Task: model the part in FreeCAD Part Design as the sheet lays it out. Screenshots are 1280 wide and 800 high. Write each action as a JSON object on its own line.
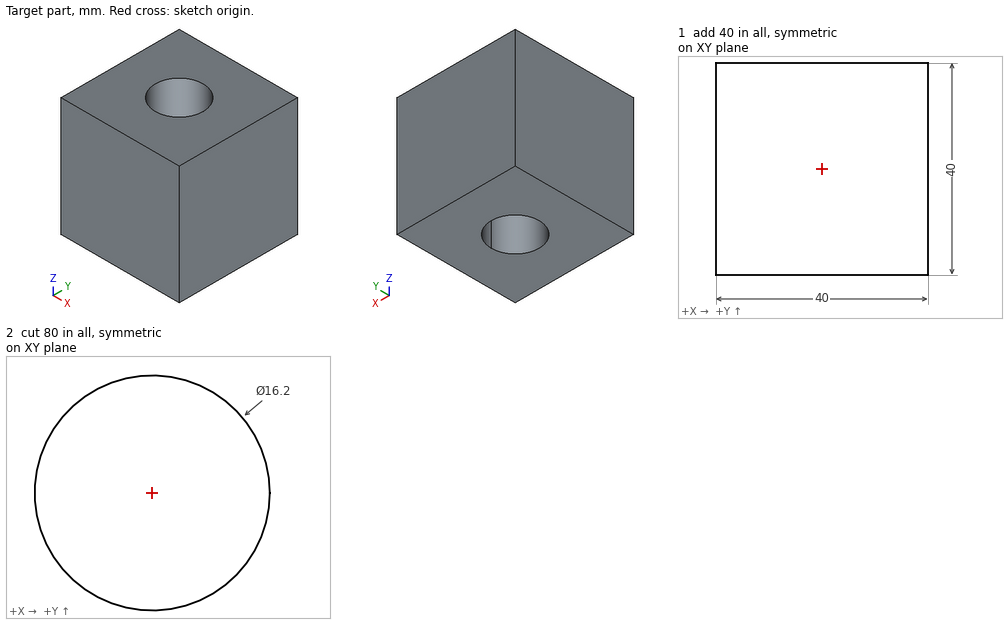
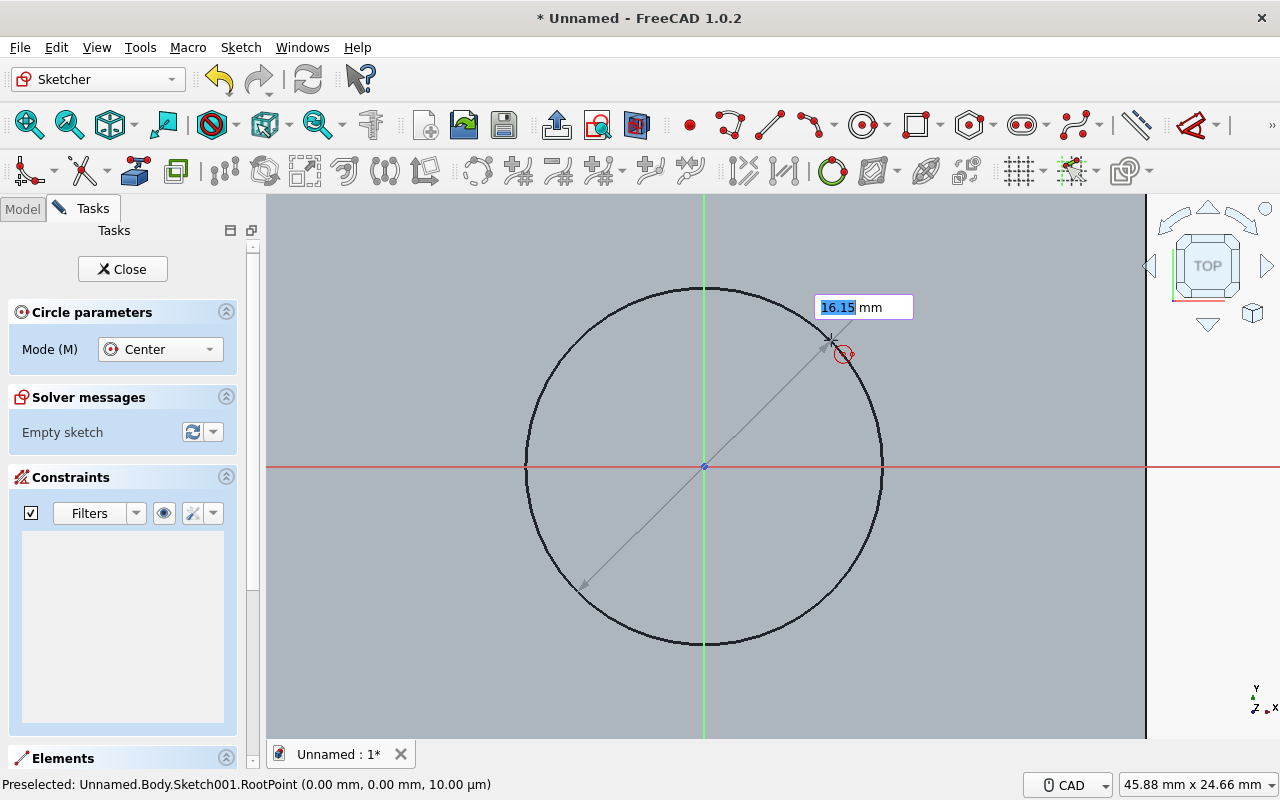
{"action": "type", "text": "16.2"}
{"action": "key", "text": "Return"}
{"action": "key", "text": "Escape"}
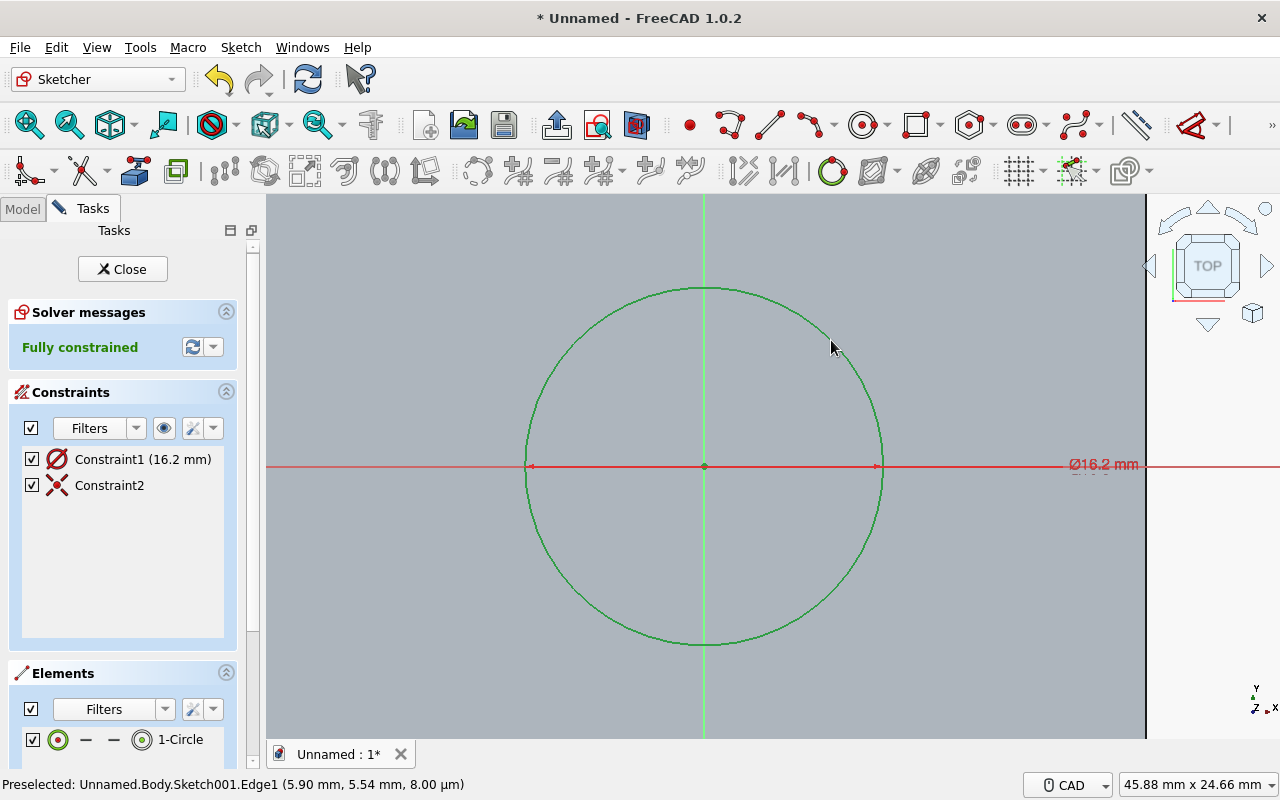
{"action": "left_click", "coordinate": [123, 269]}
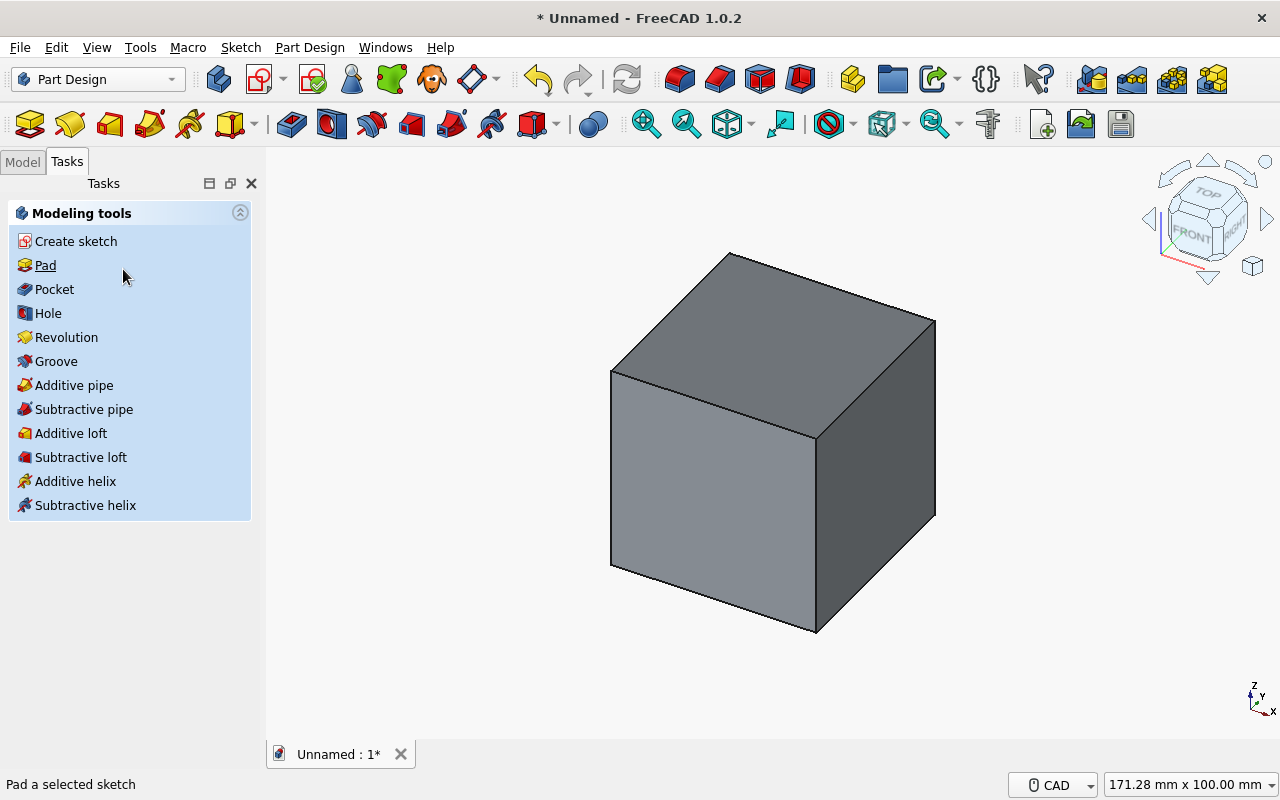
{"action": "left_click", "coordinate": [292, 124]}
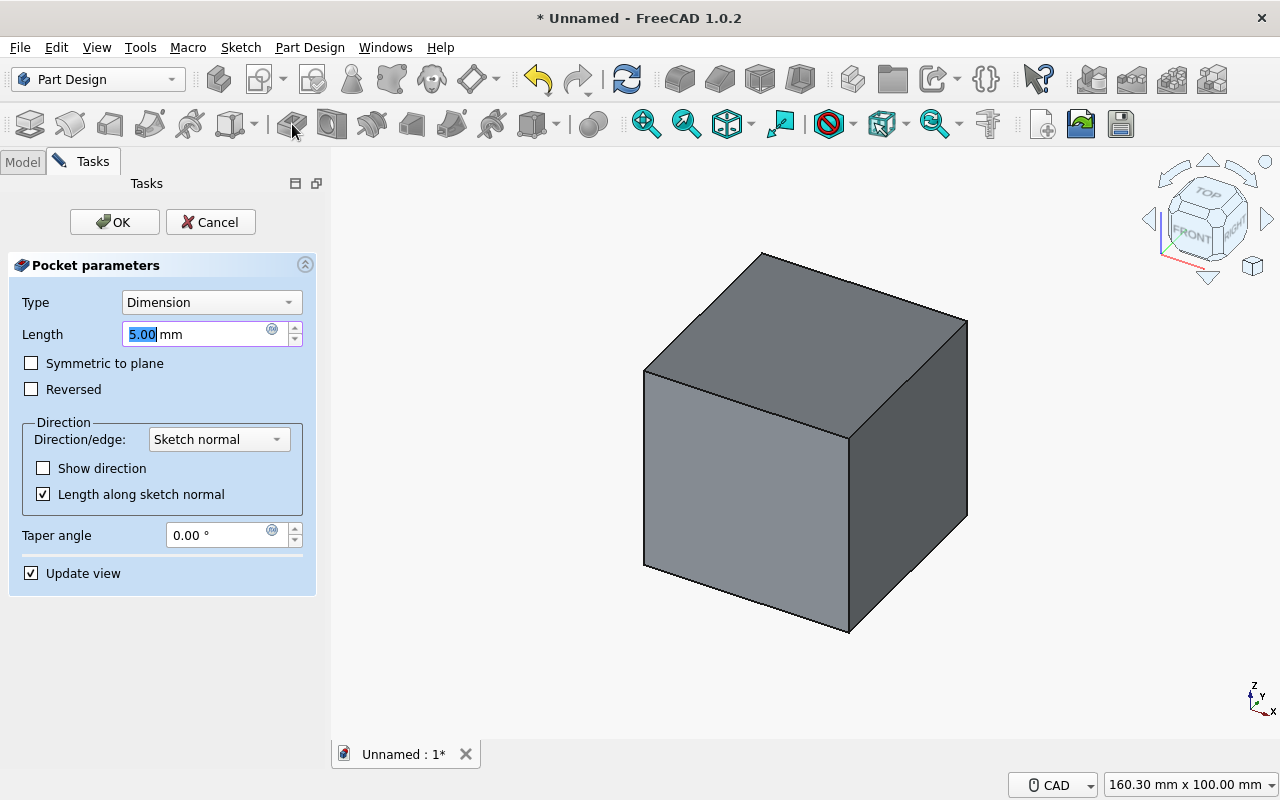
{"action": "type", "text": "80"}
{"action": "key", "text": "Tab"}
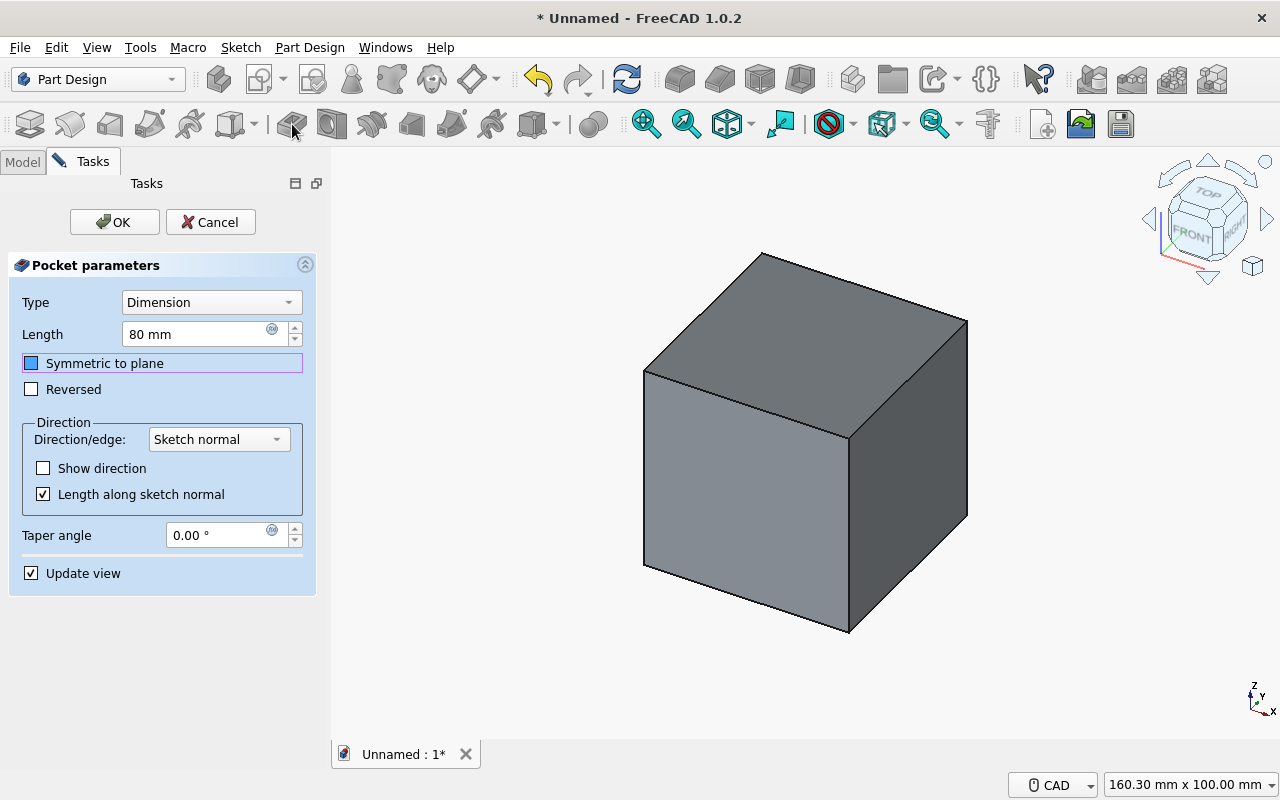
{"action": "left_click", "coordinate": [30, 363]}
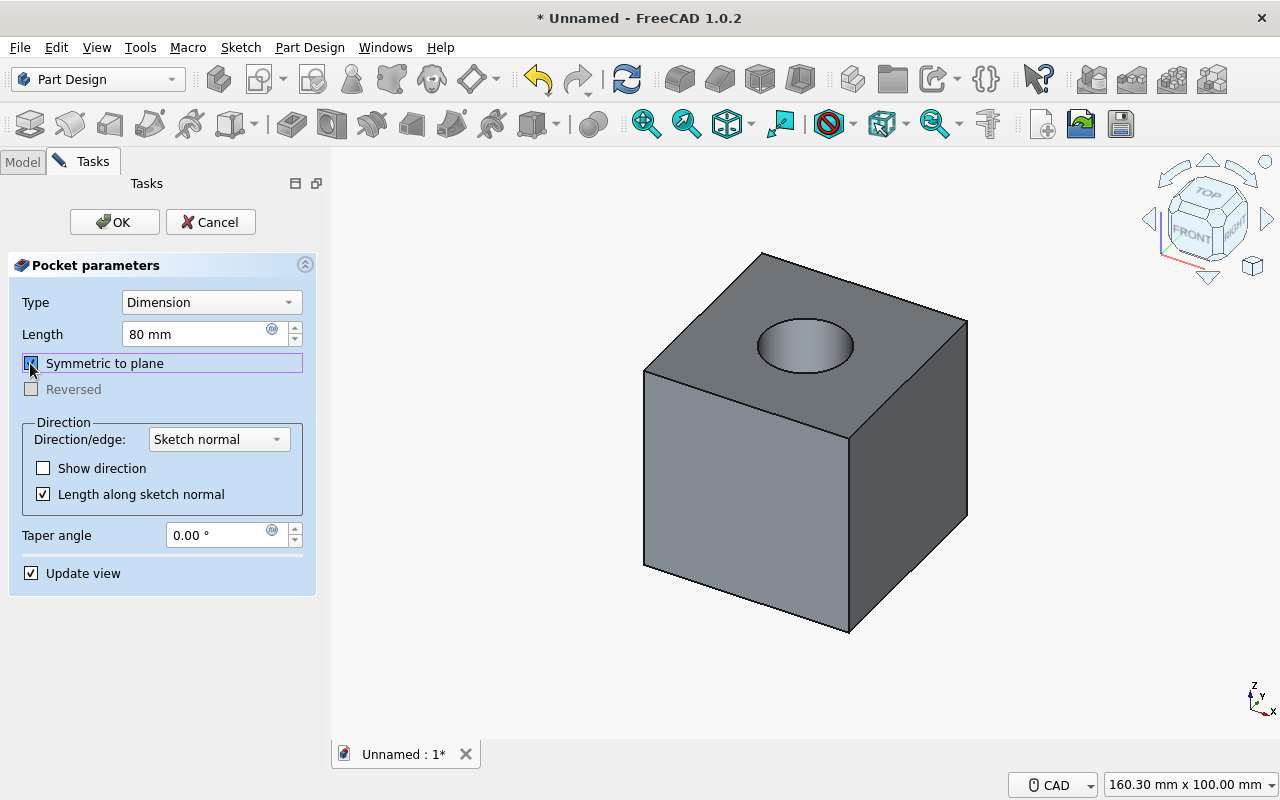
{"action": "left_click", "coordinate": [115, 222]}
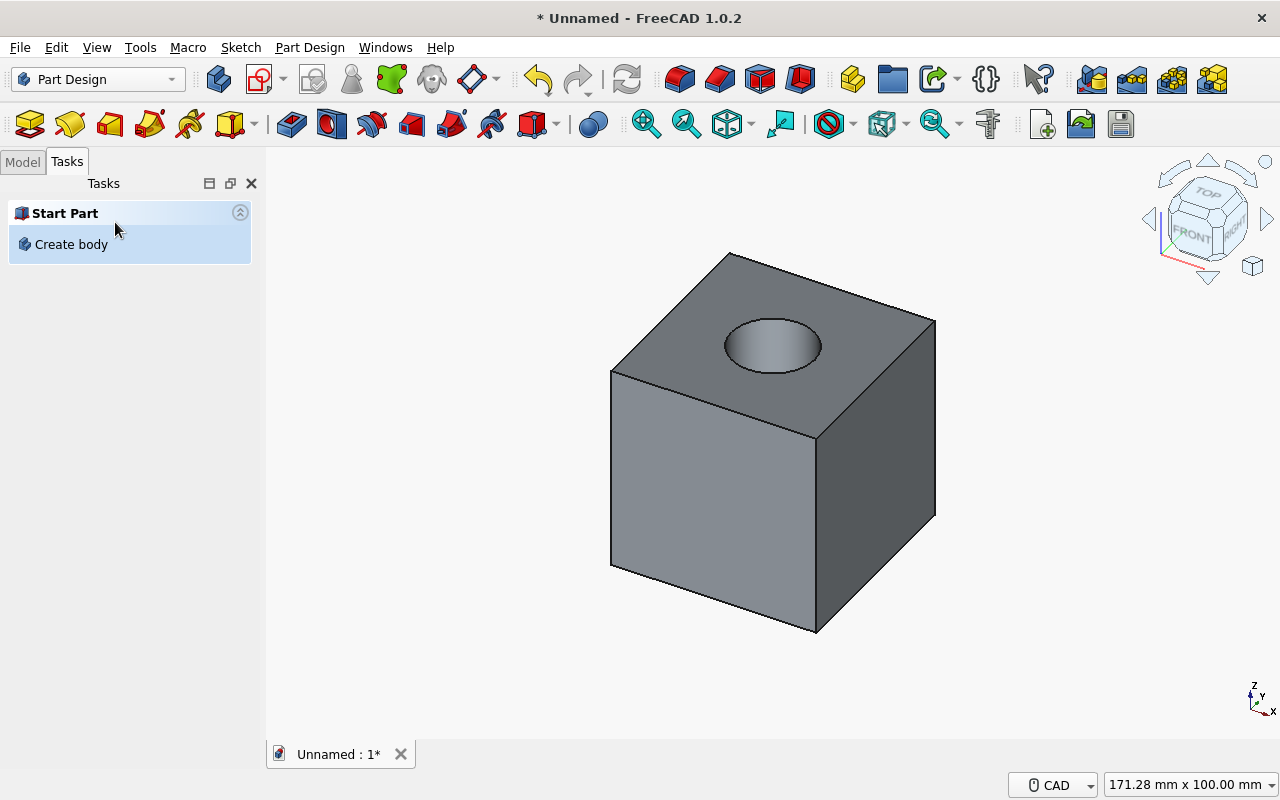
{"action": "key", "text": "0"}